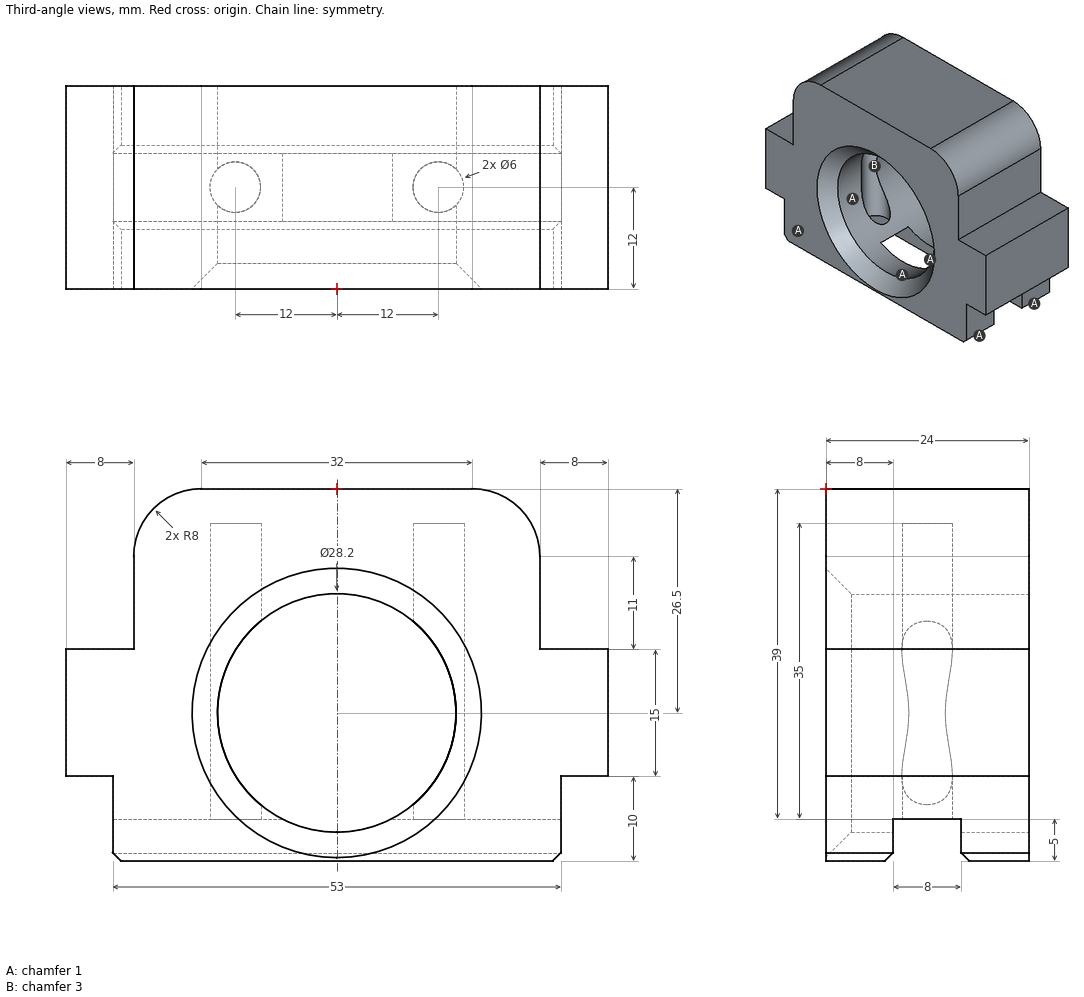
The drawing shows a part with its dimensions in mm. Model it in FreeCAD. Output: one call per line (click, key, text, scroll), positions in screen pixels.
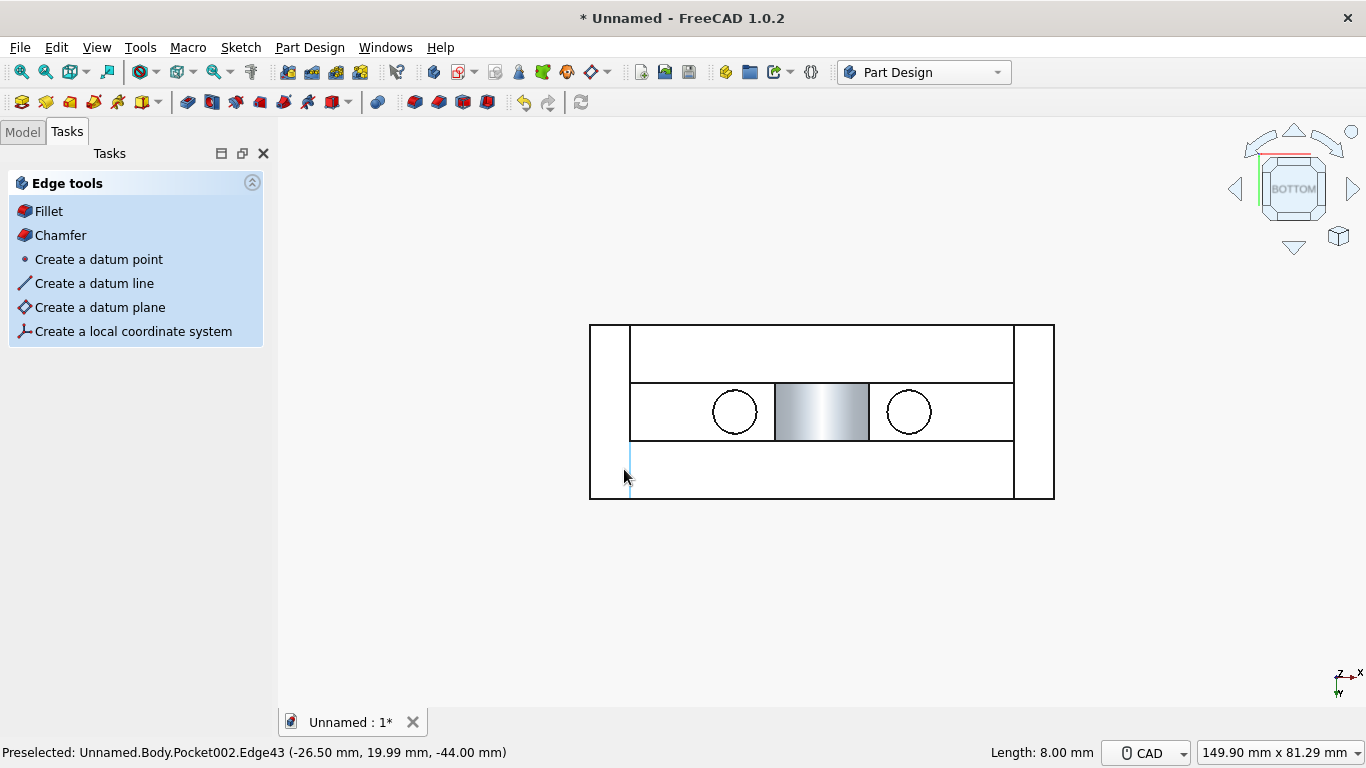
click(1014, 469, ctrl)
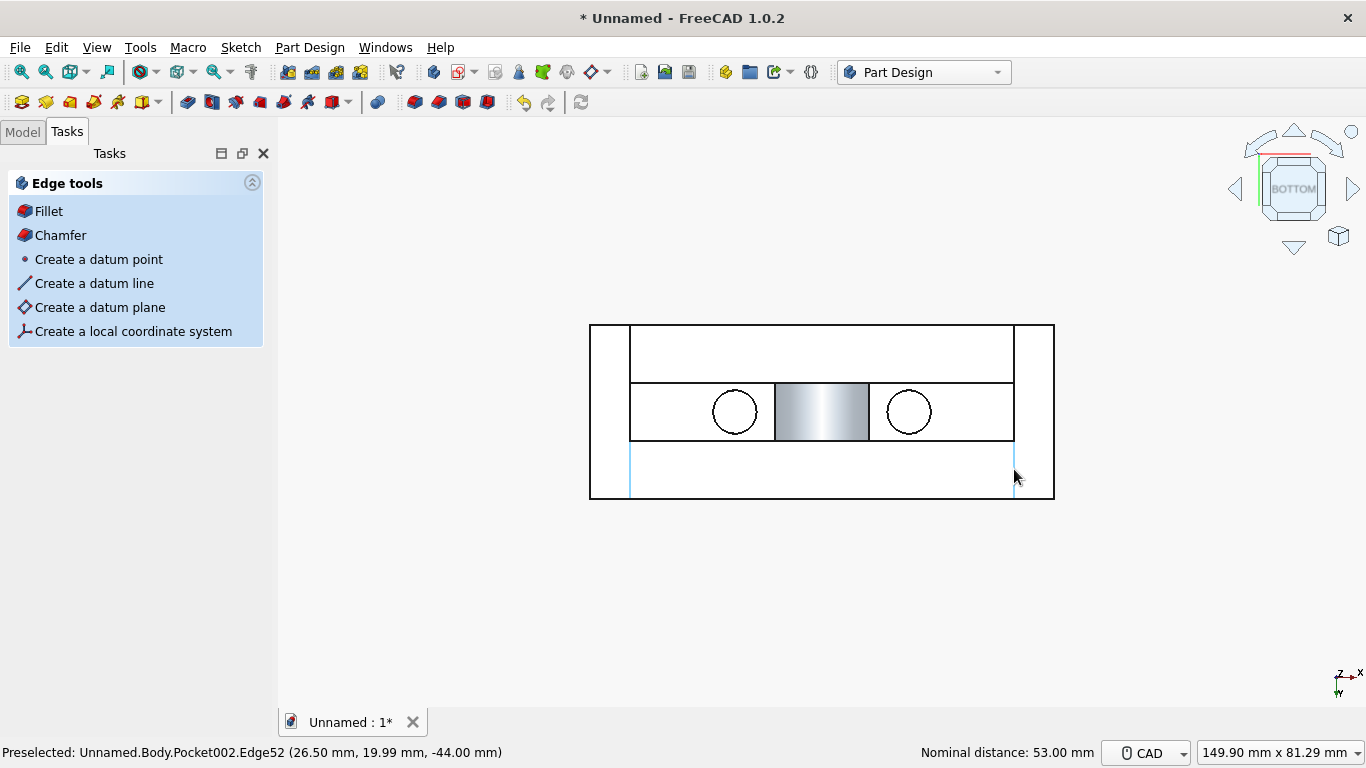
click(630, 353, ctrl)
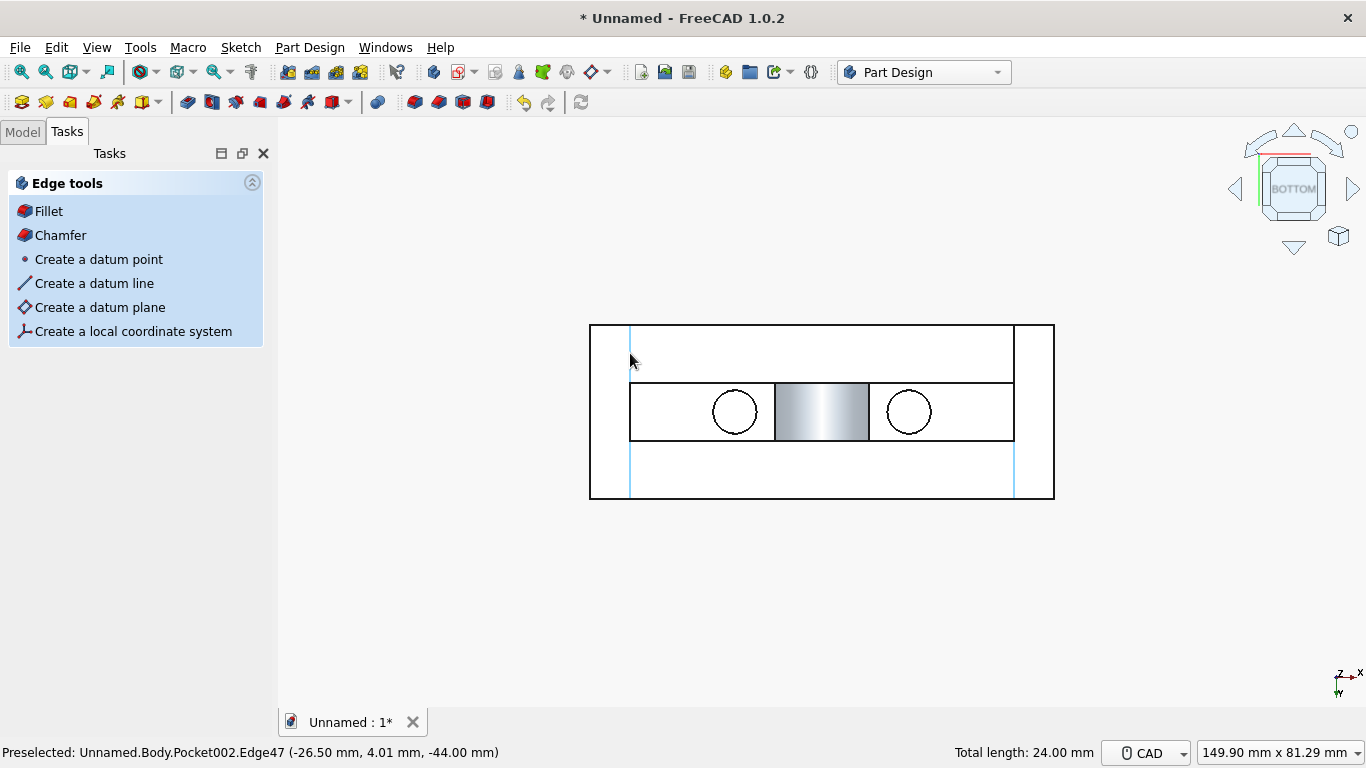
click(1014, 353, ctrl)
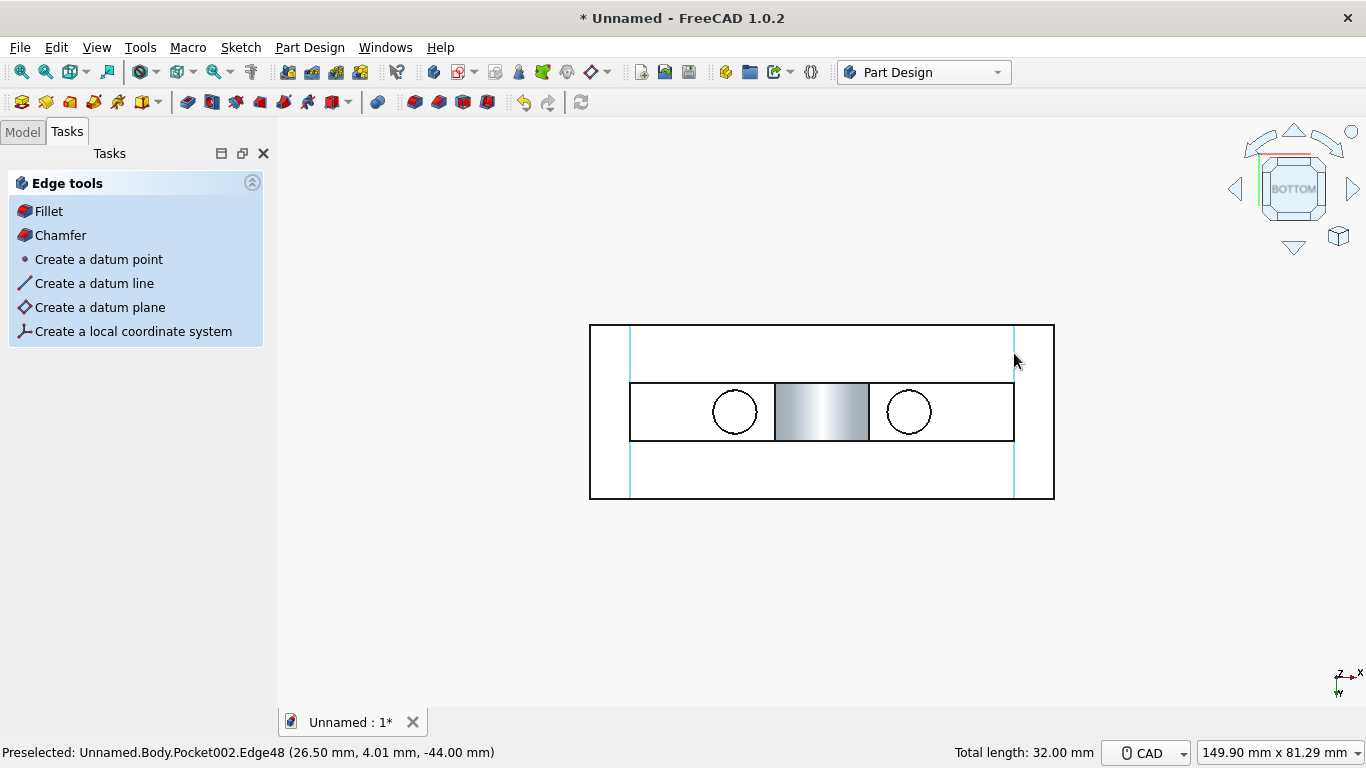
click(822, 440, ctrl)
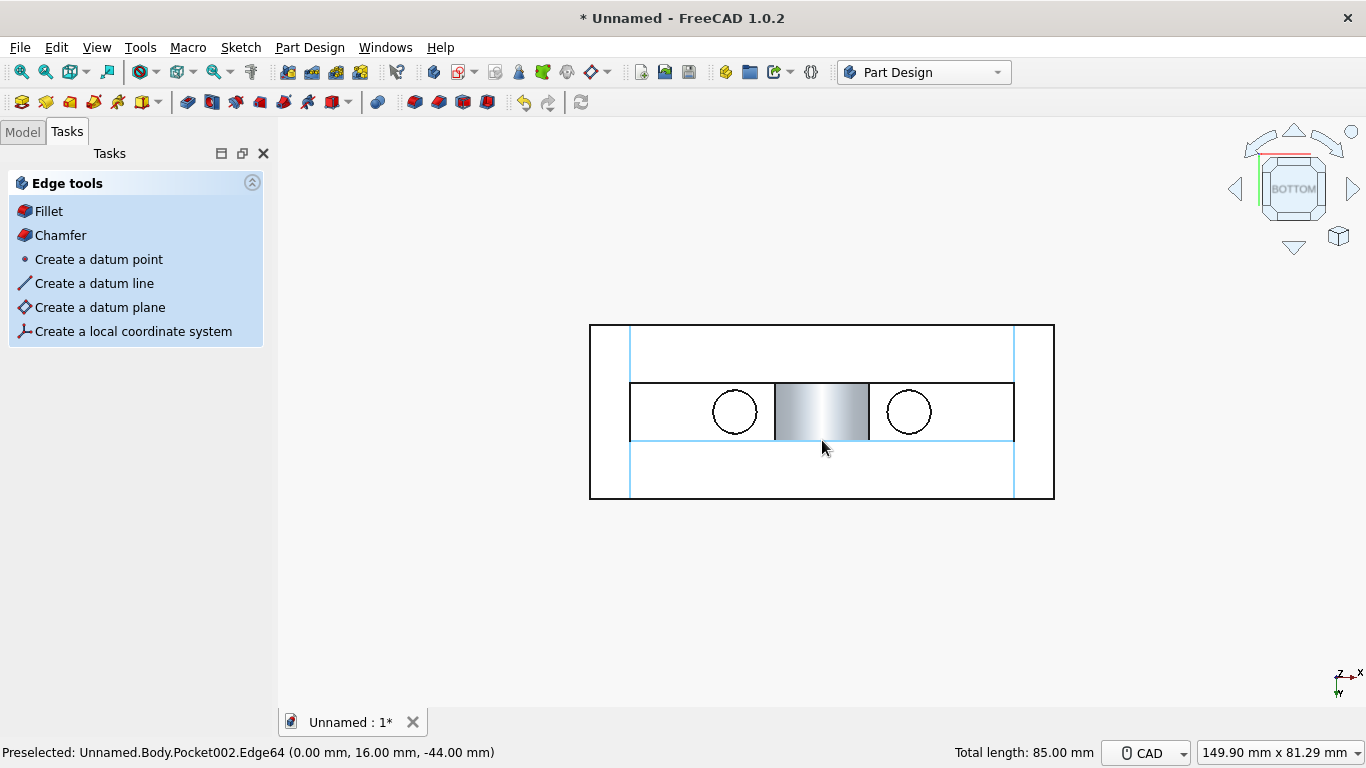
key(0)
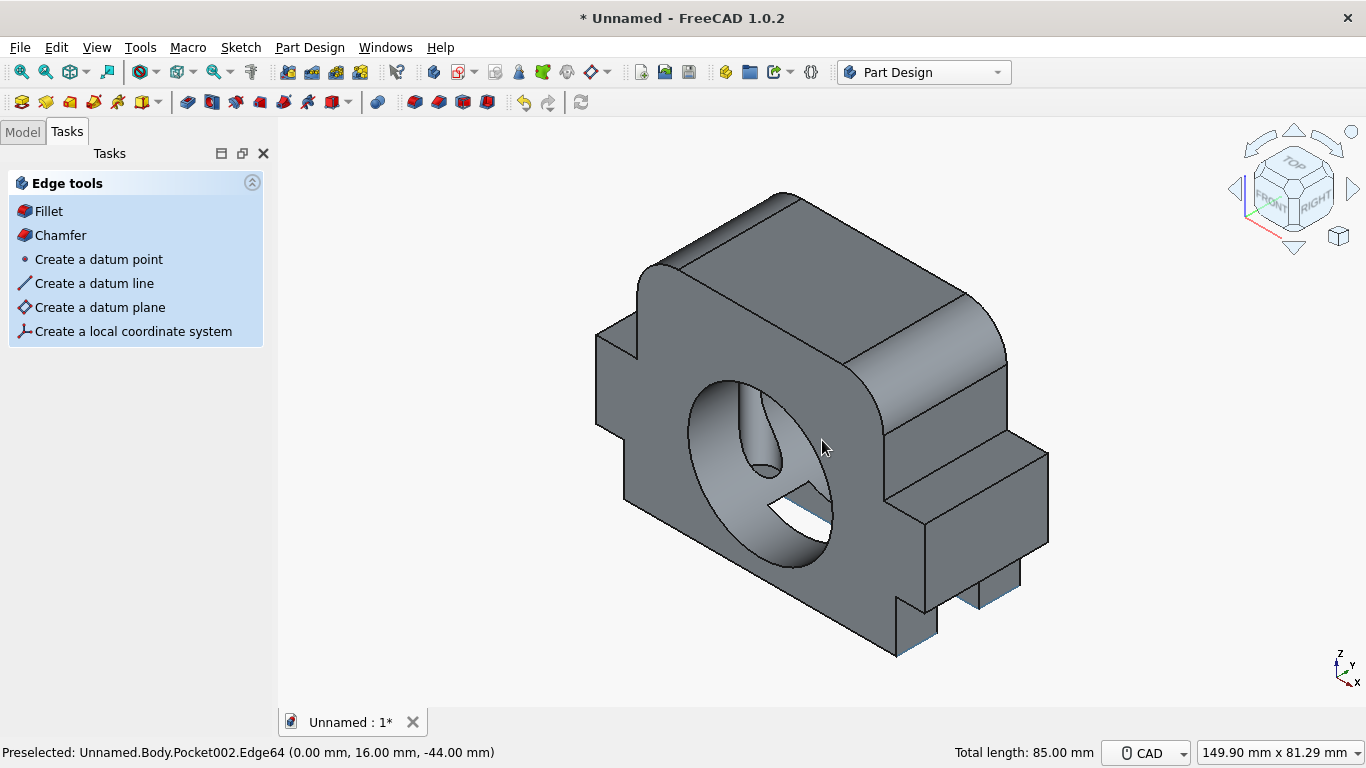
key(2)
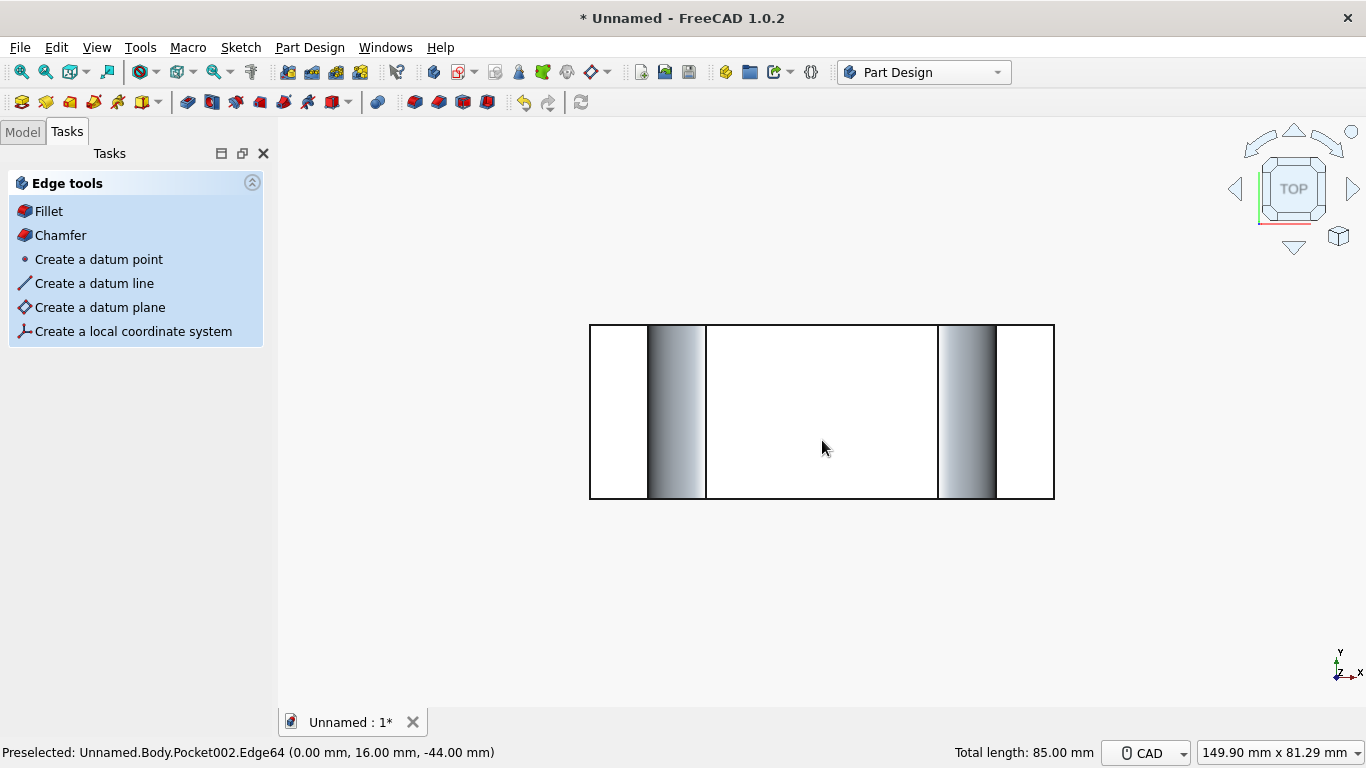
key(v)
key(f)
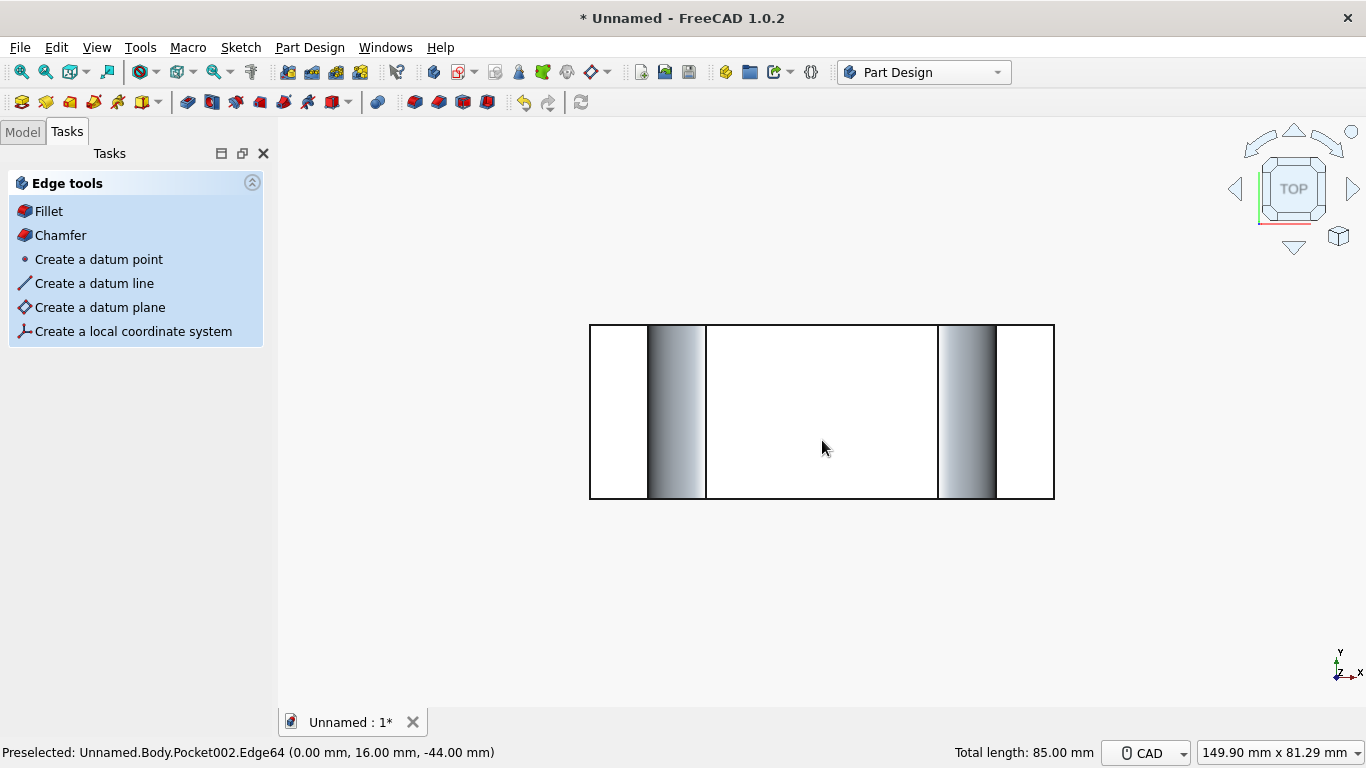
key(1)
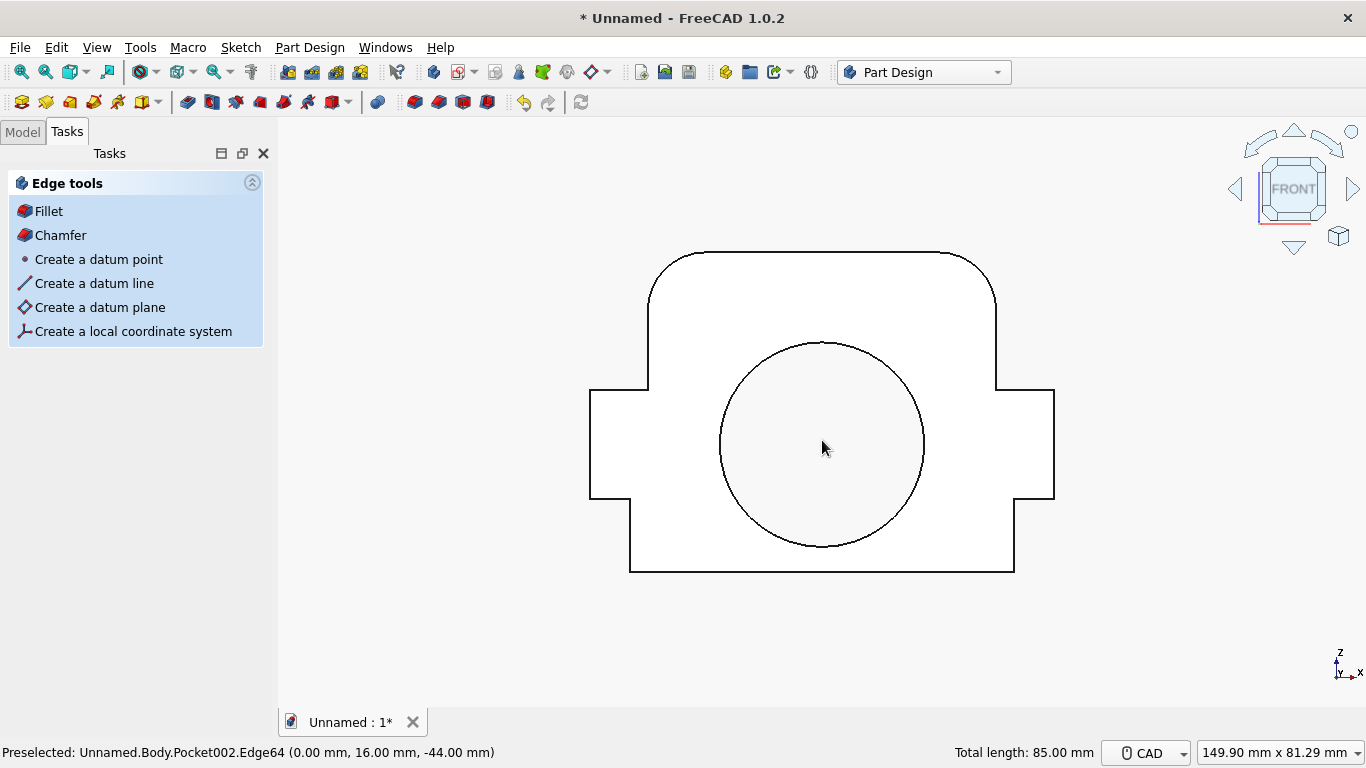
key(3)